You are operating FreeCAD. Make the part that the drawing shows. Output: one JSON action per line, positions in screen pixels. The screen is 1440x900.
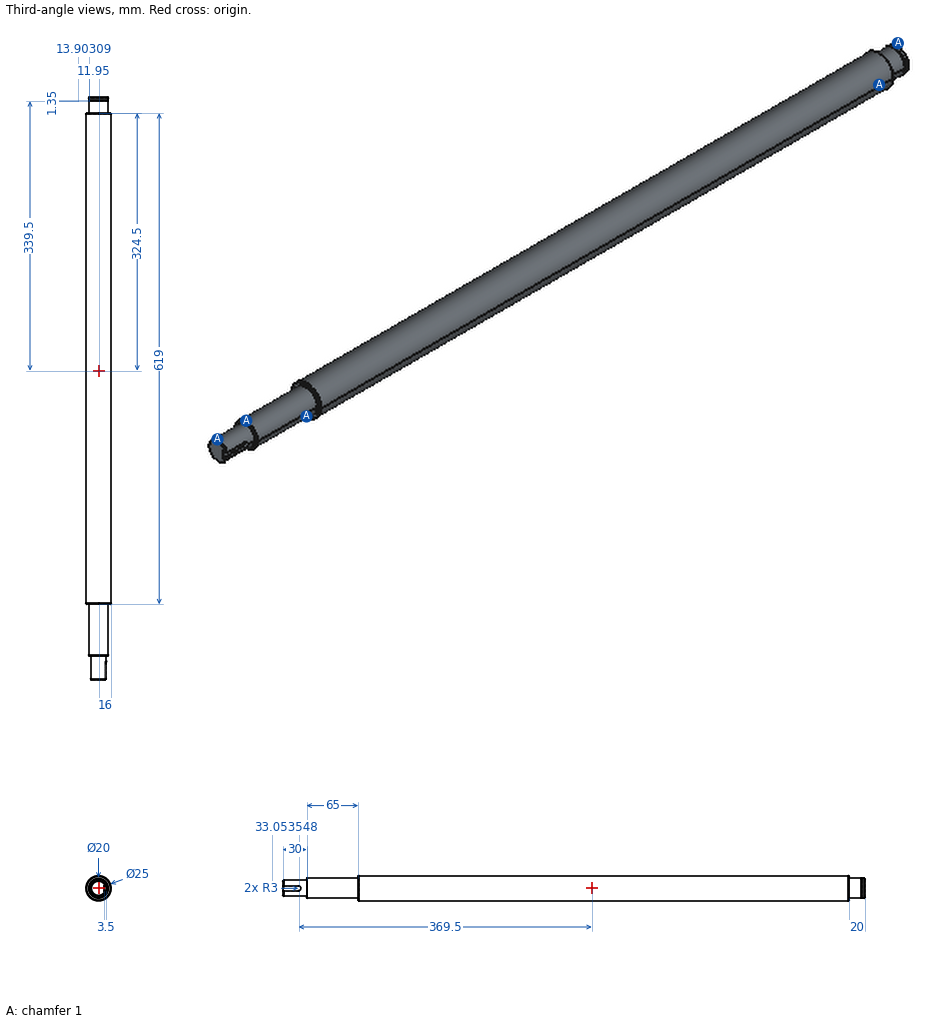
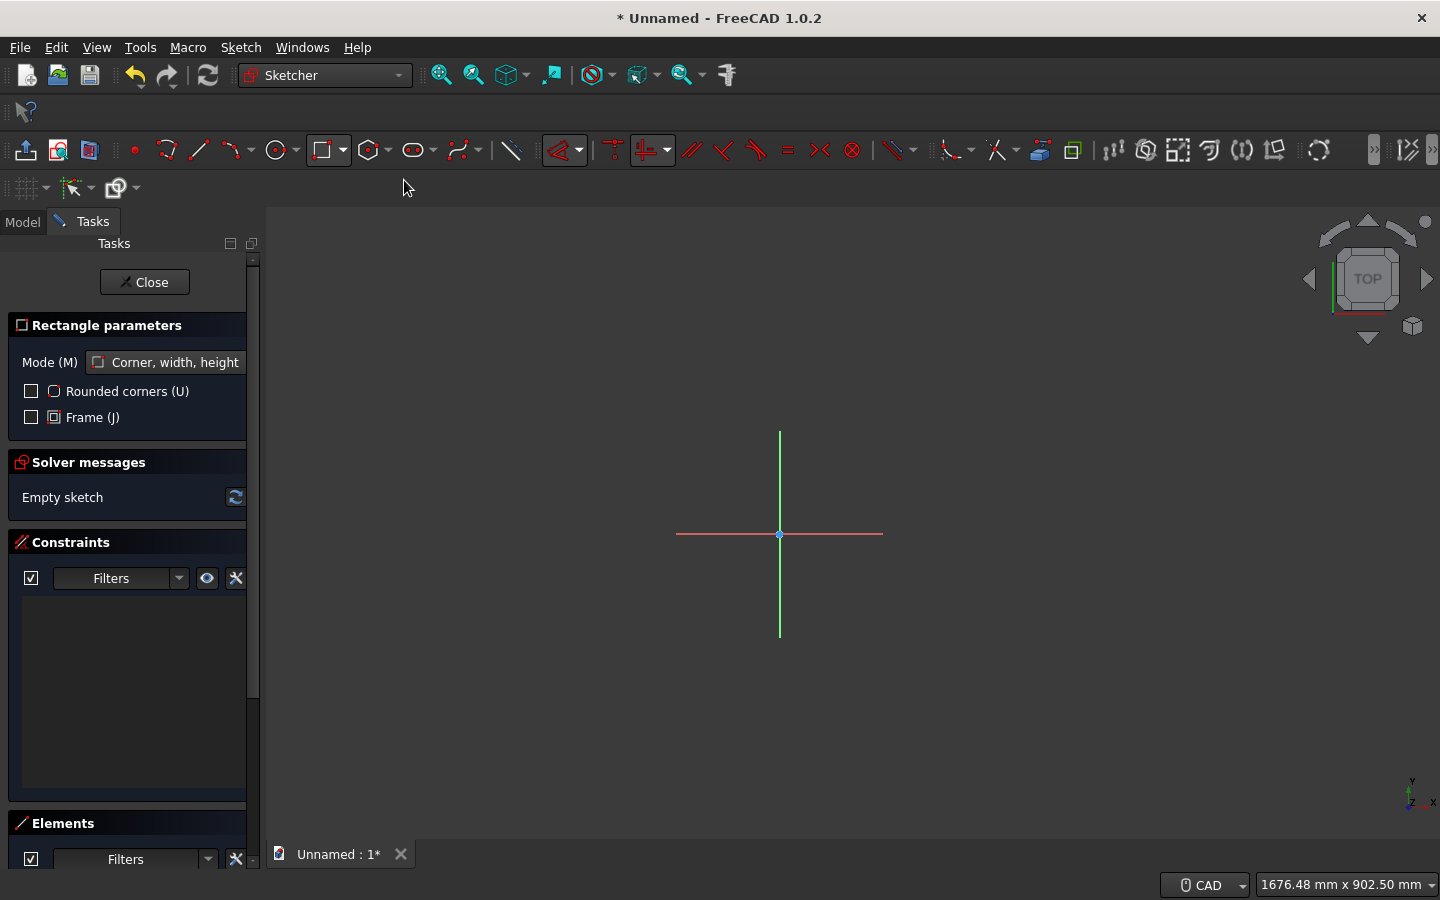
{"action": "scroll", "coordinate": [780, 307], "scroll_direction": "up", "scroll_amount": 2}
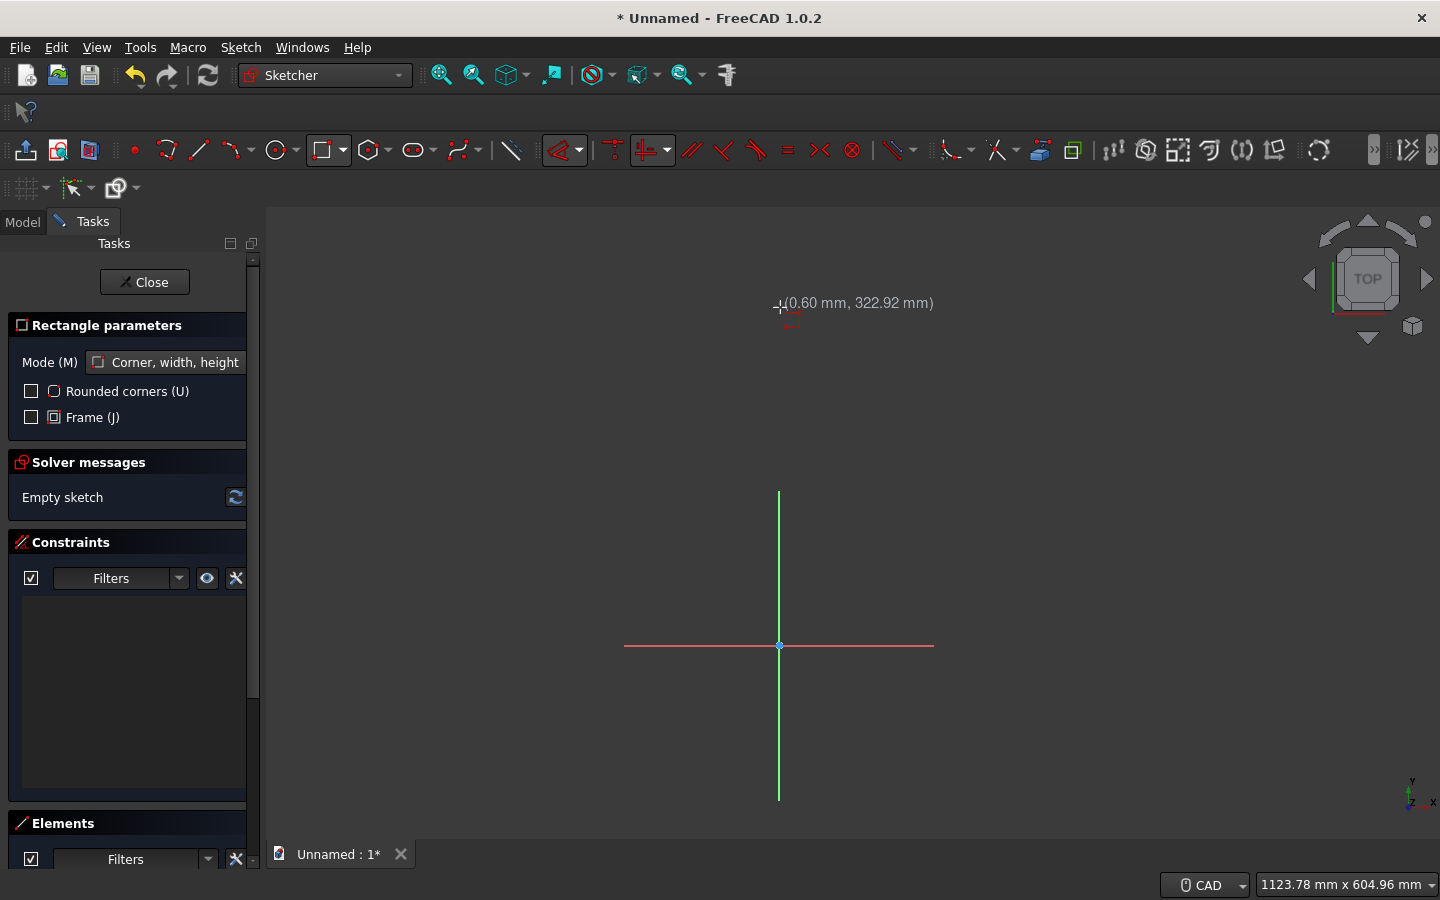
{"action": "left_click", "coordinate": [779, 307]}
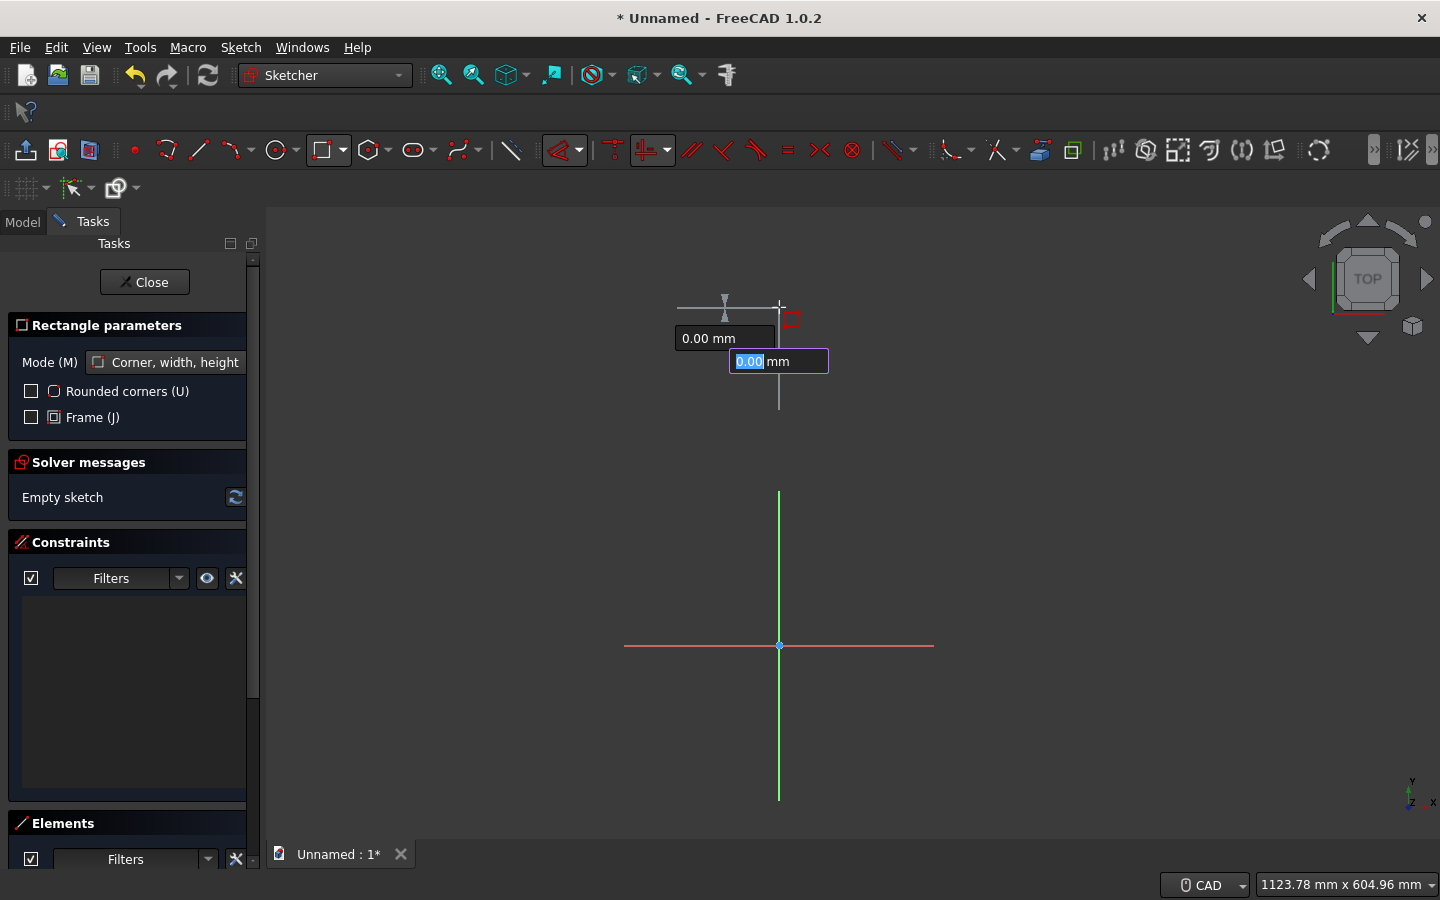
{"action": "scroll", "coordinate": [778, 305], "scroll_direction": "down", "scroll_amount": 2}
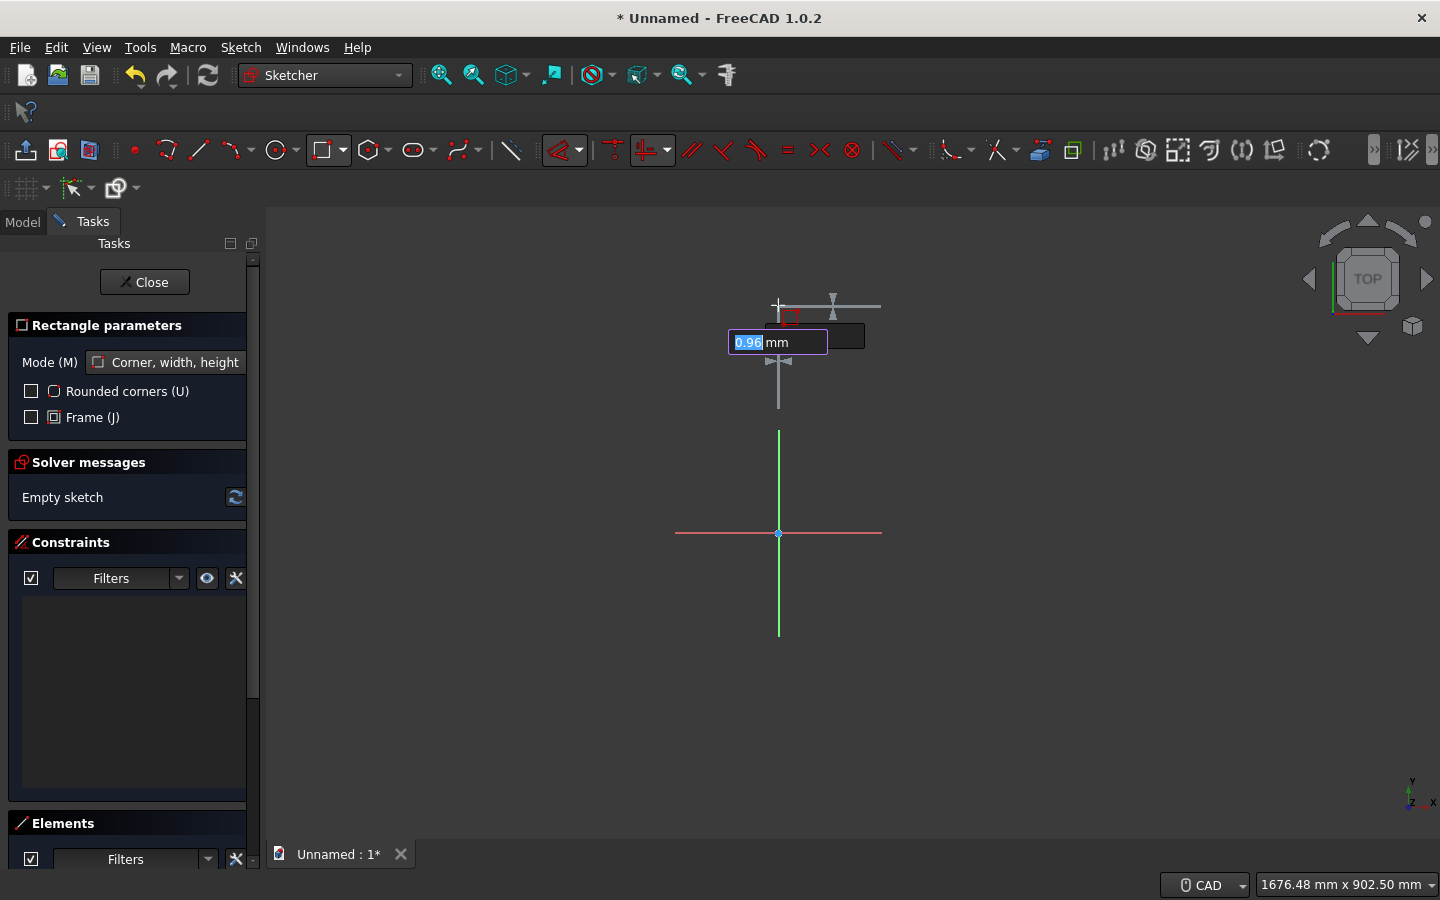
{"action": "scroll", "coordinate": [790, 740], "scroll_direction": "up", "scroll_amount": 2}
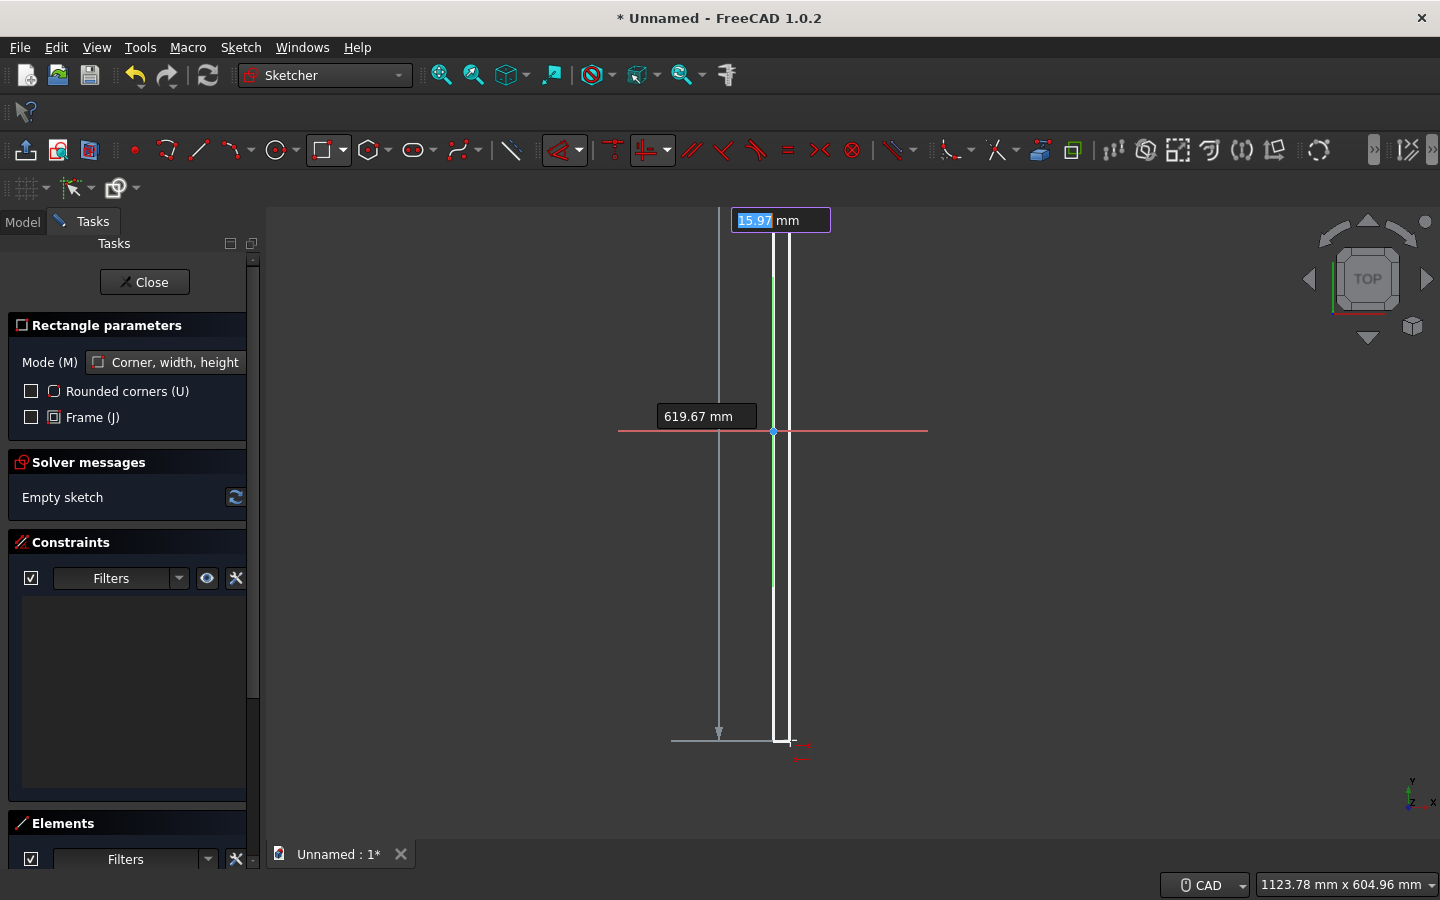
{"action": "left_click", "coordinate": [790, 739]}
{"action": "key", "text": "Escape"}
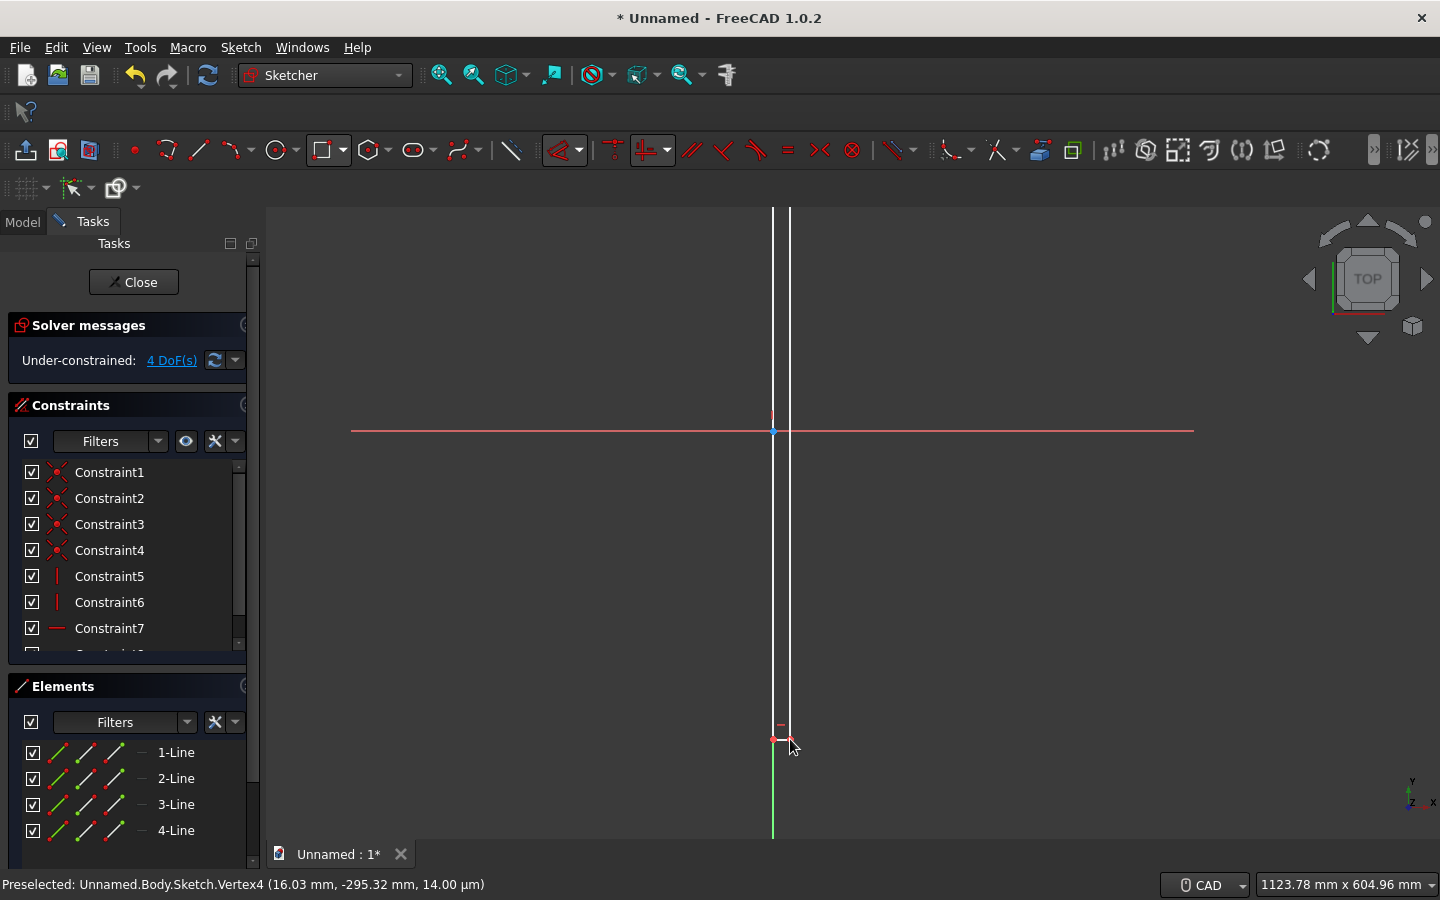
{"action": "scroll", "coordinate": [790, 741], "scroll_direction": "down", "scroll_amount": 2}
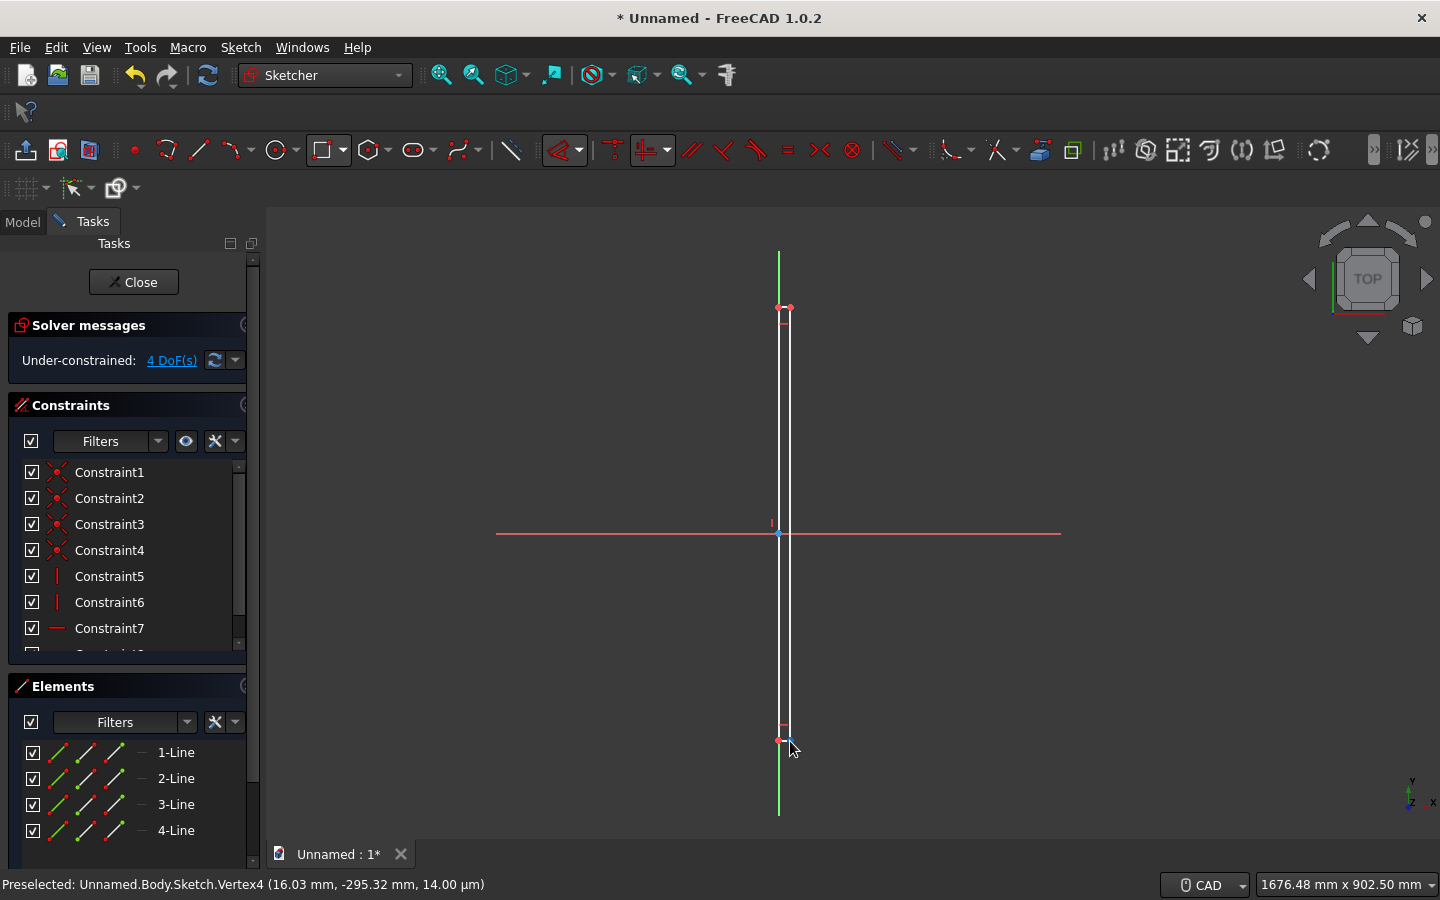
{"action": "left_click", "coordinate": [779, 307]}